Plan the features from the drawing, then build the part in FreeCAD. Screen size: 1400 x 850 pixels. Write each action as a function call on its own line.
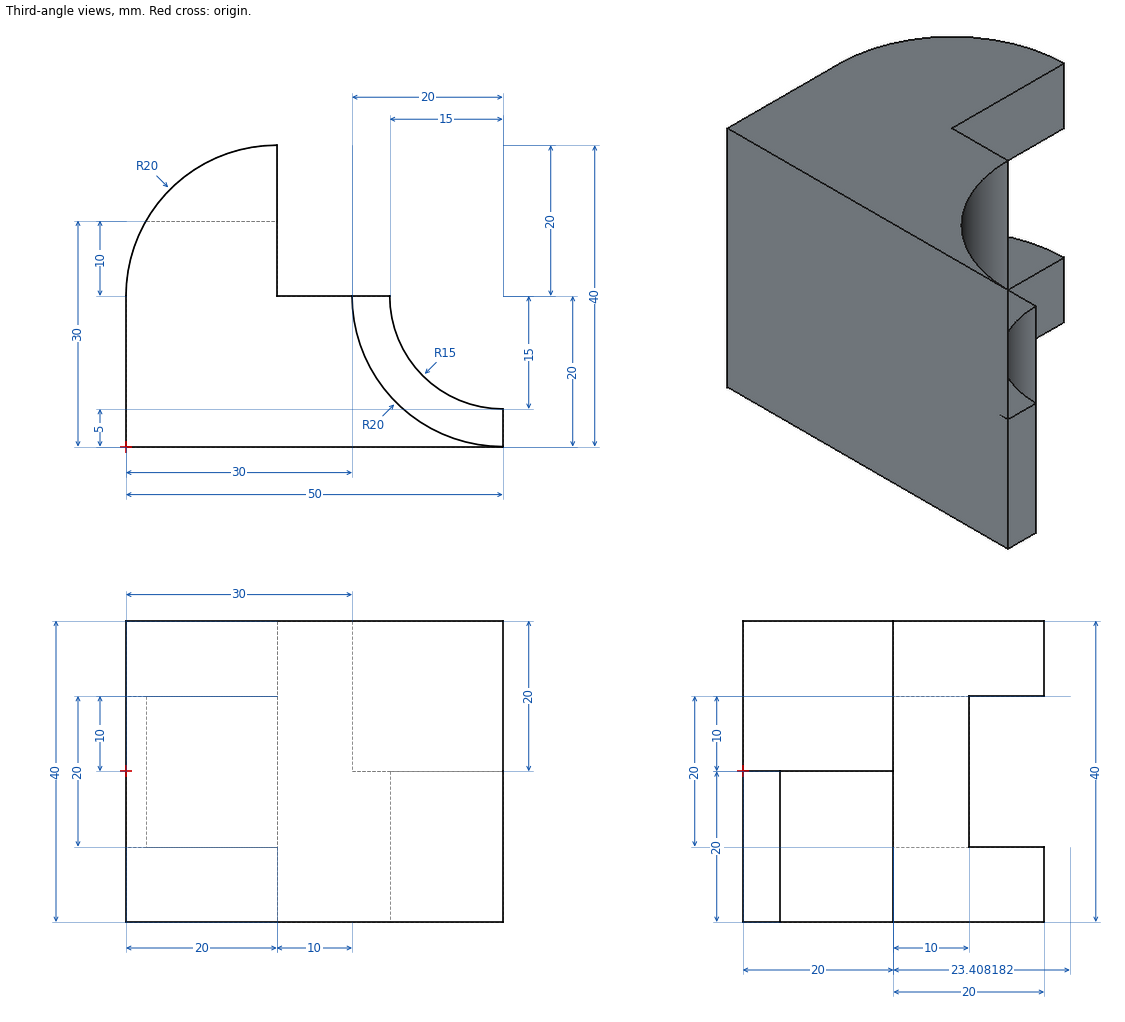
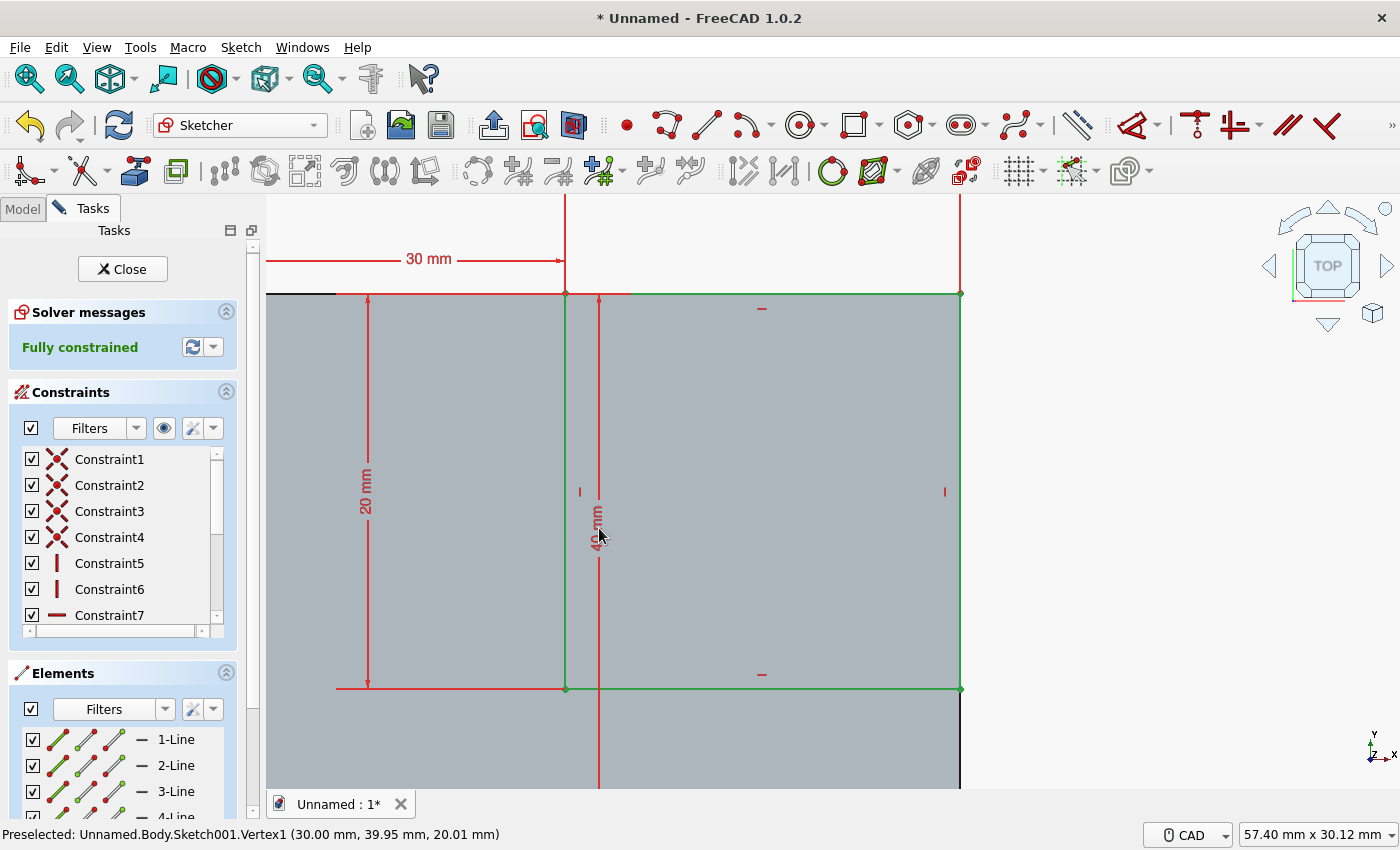
click(123, 269)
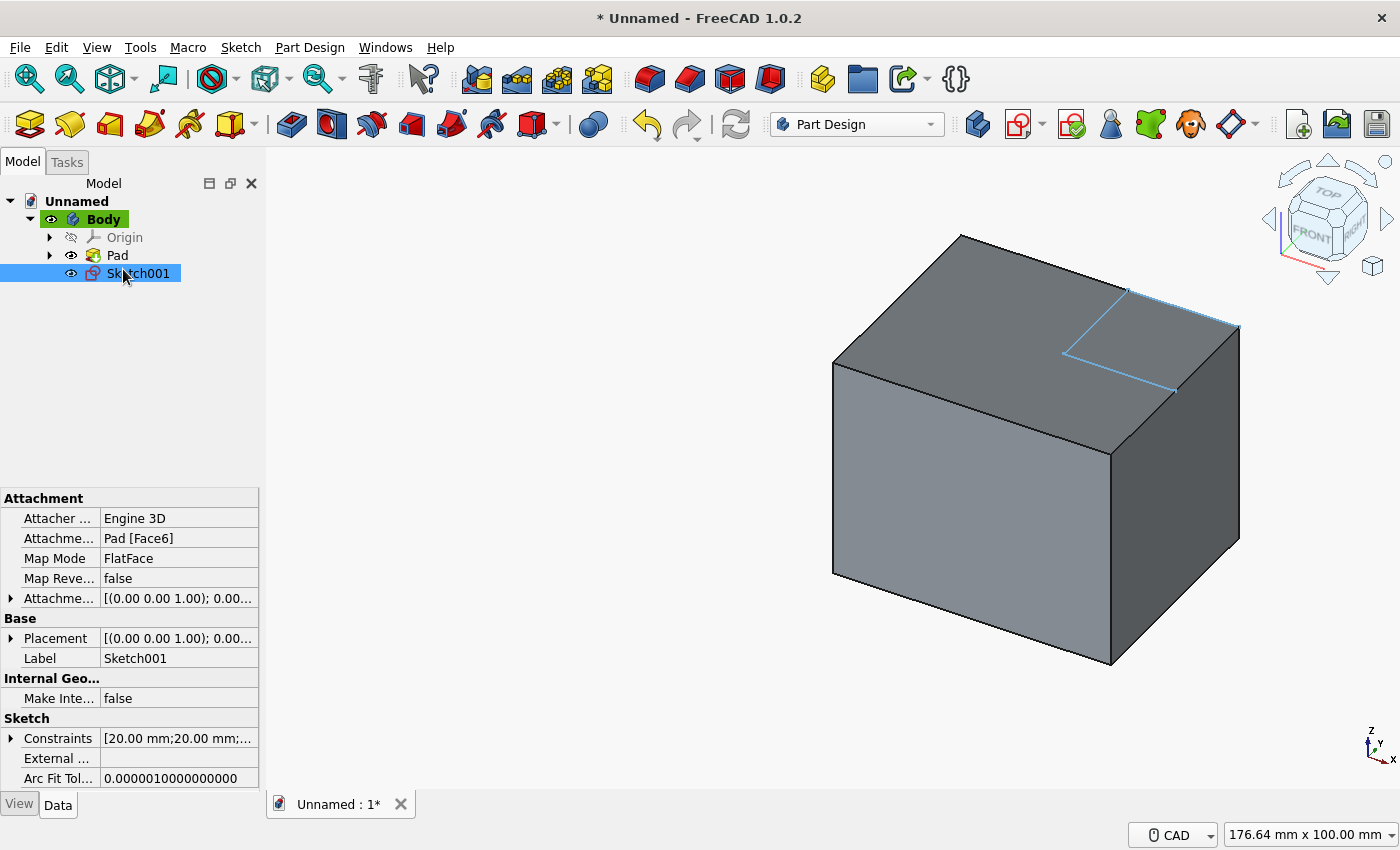
click(292, 124)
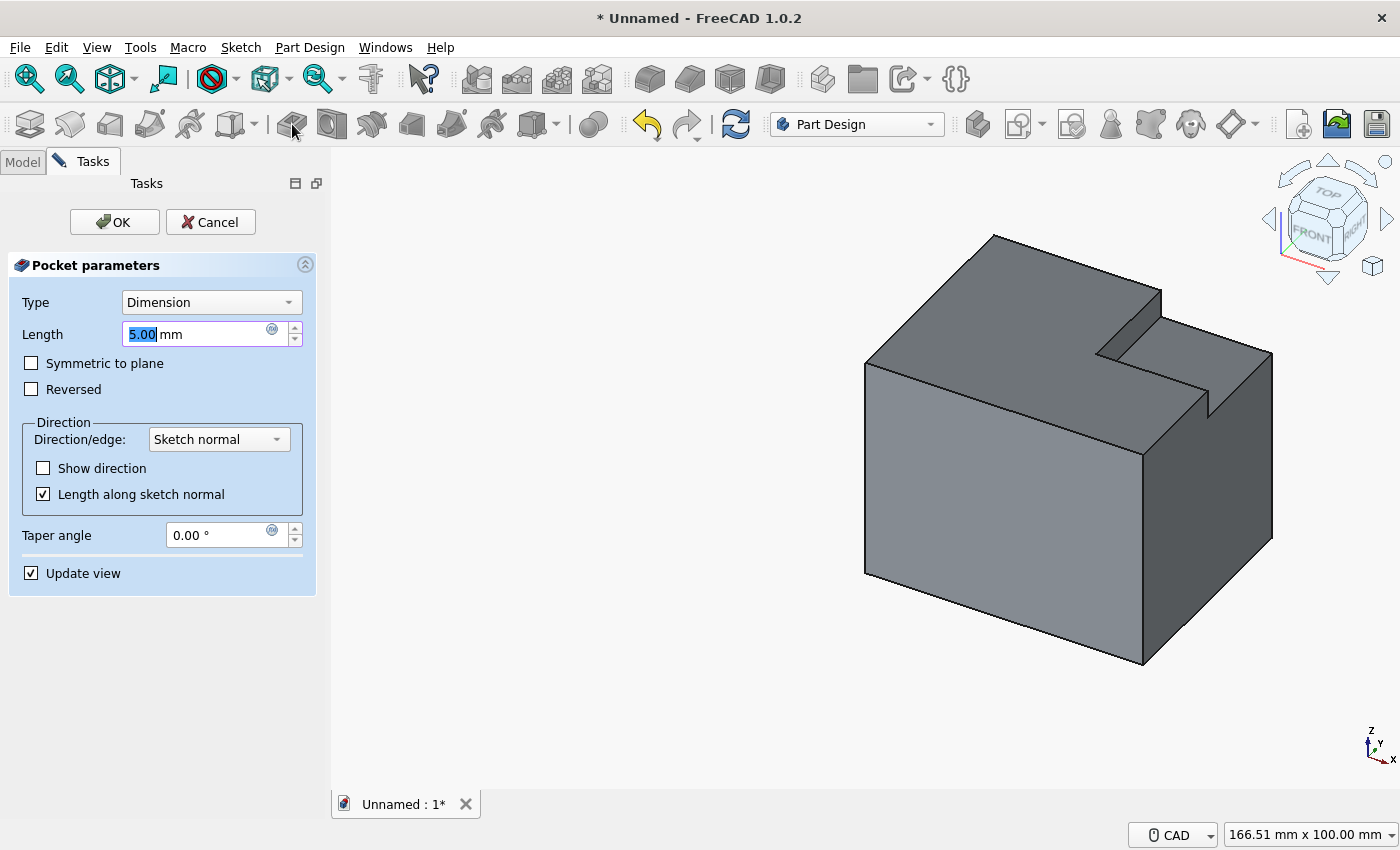
click(212, 302)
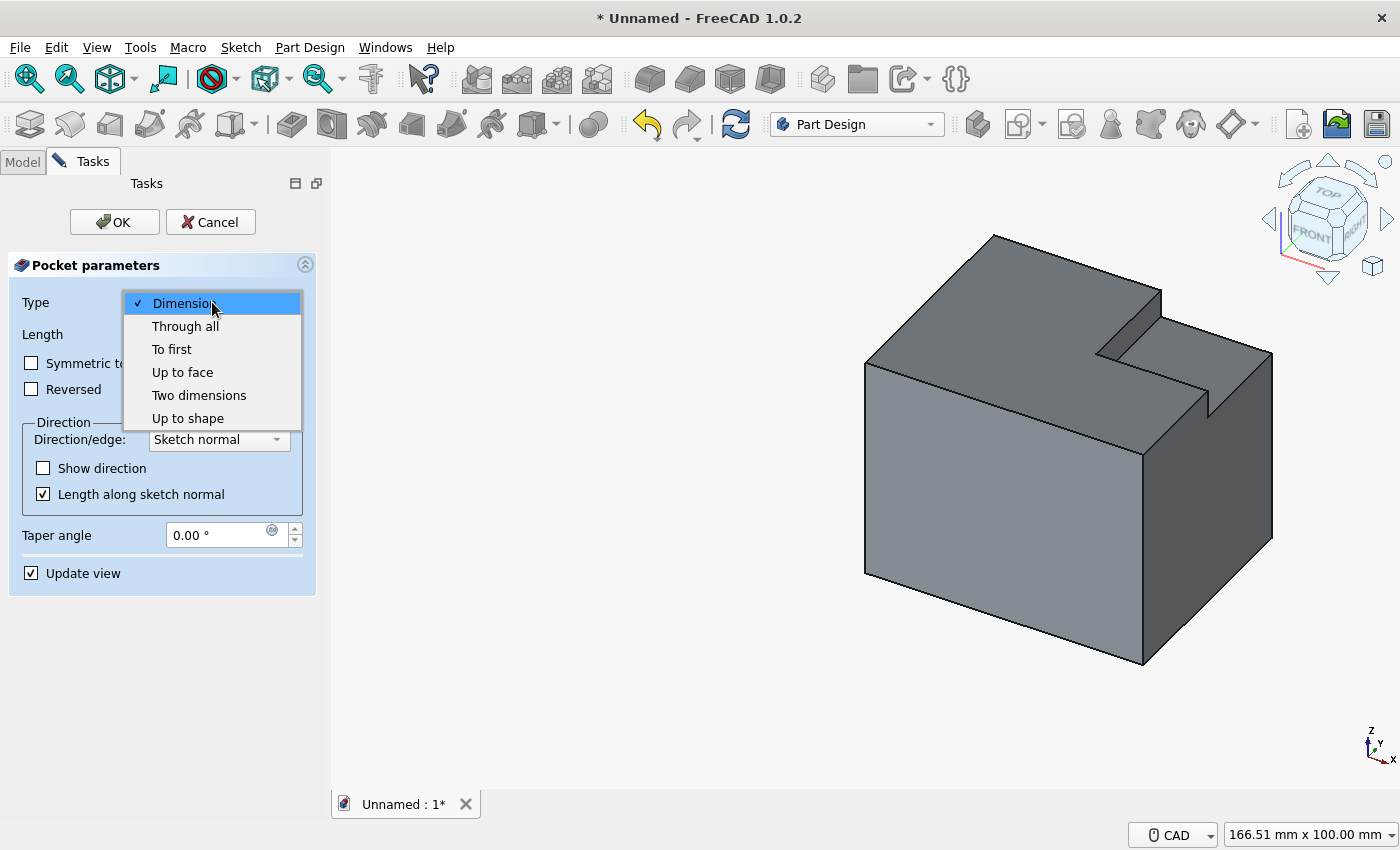
click(212, 326)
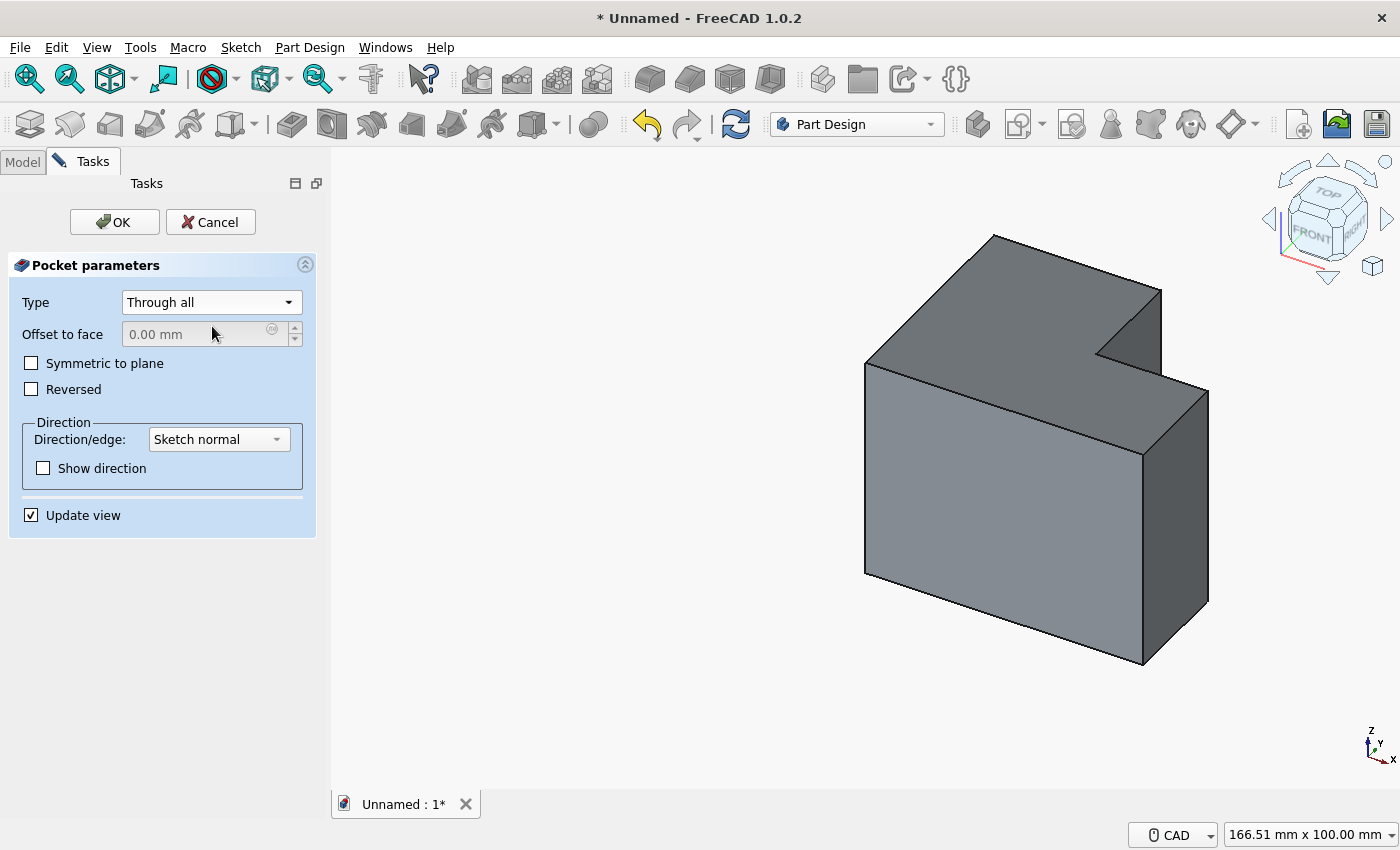
click(115, 222)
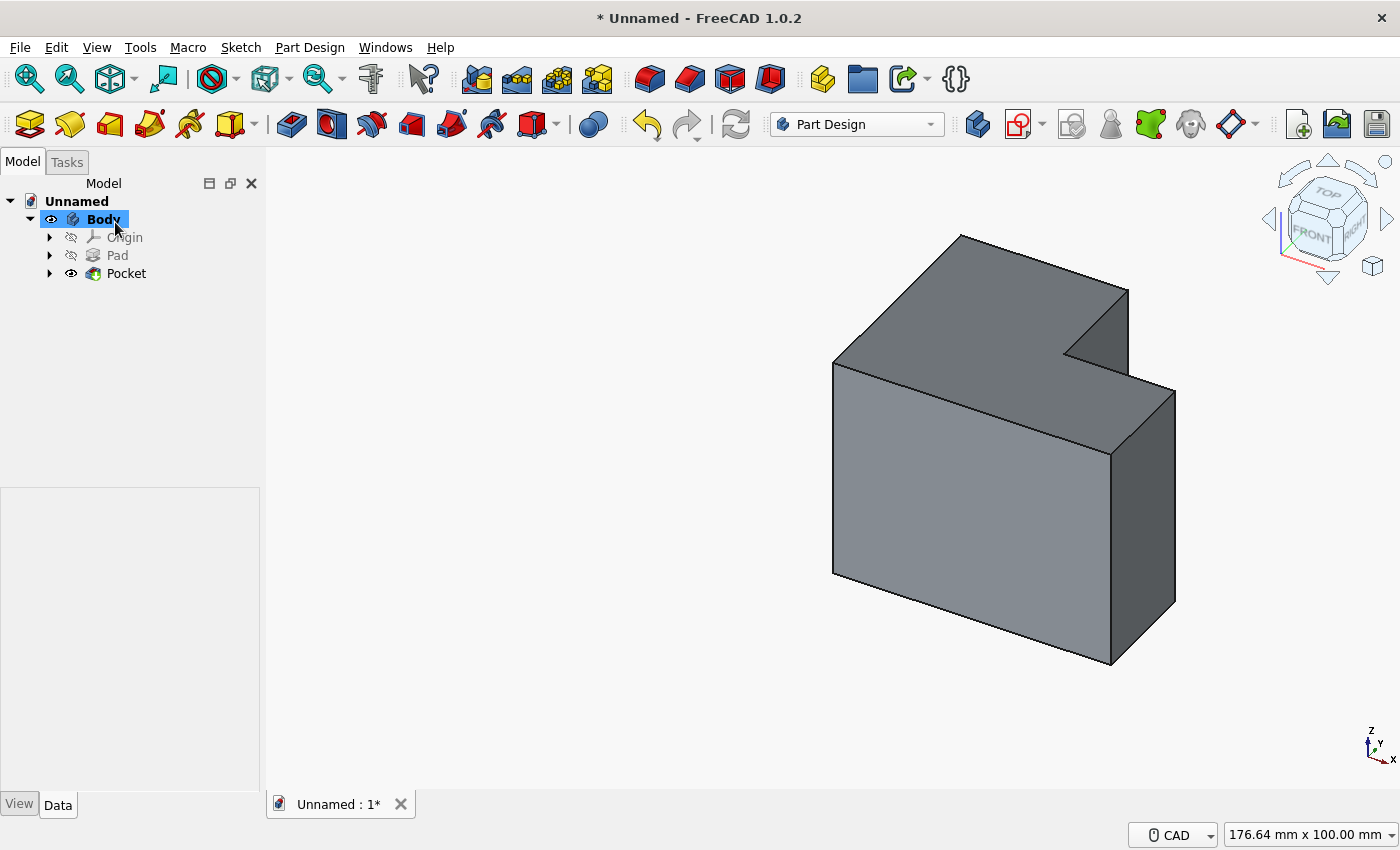
click(978, 349)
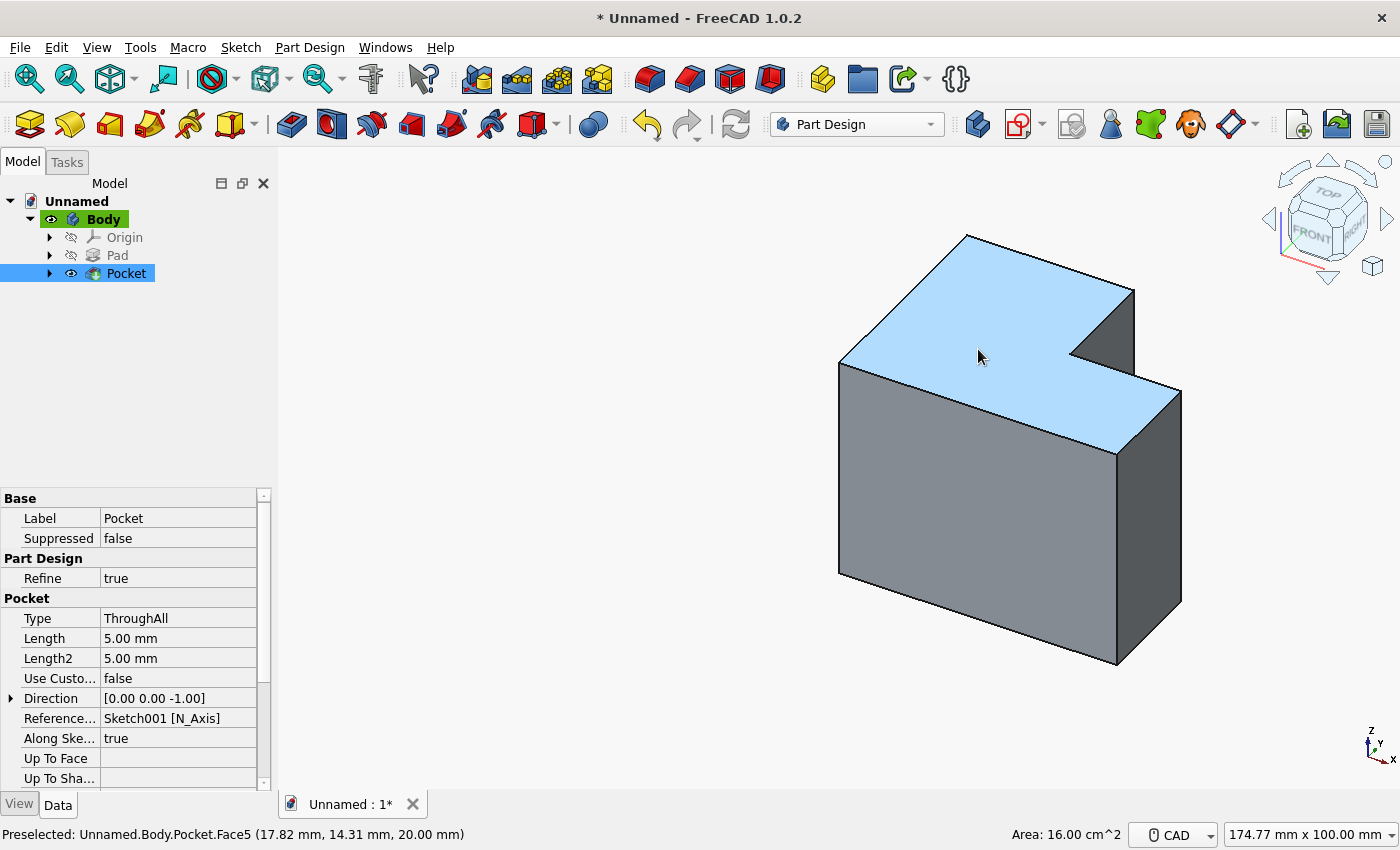
click(1018, 124)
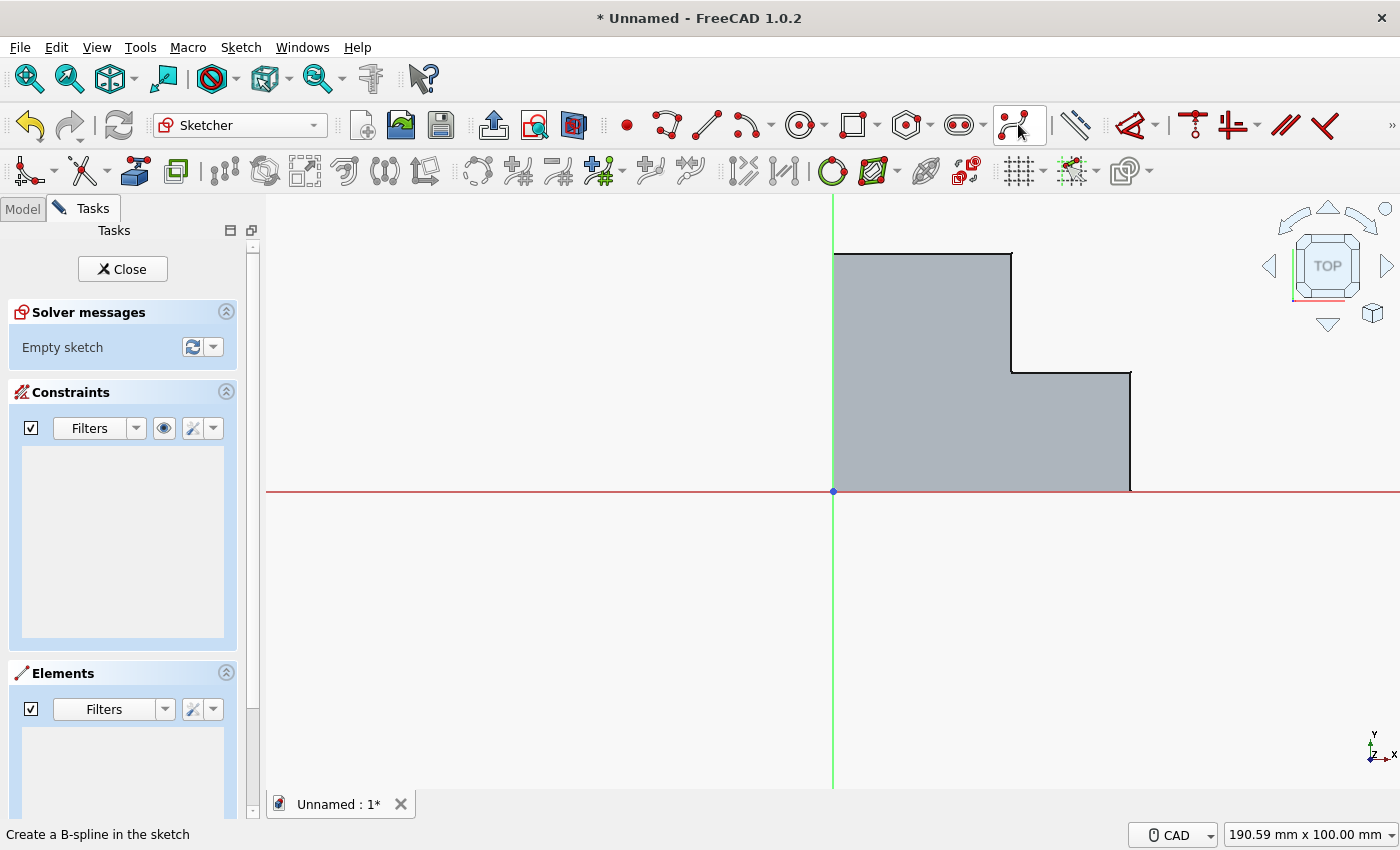
scroll(1203, 406, up, 6)